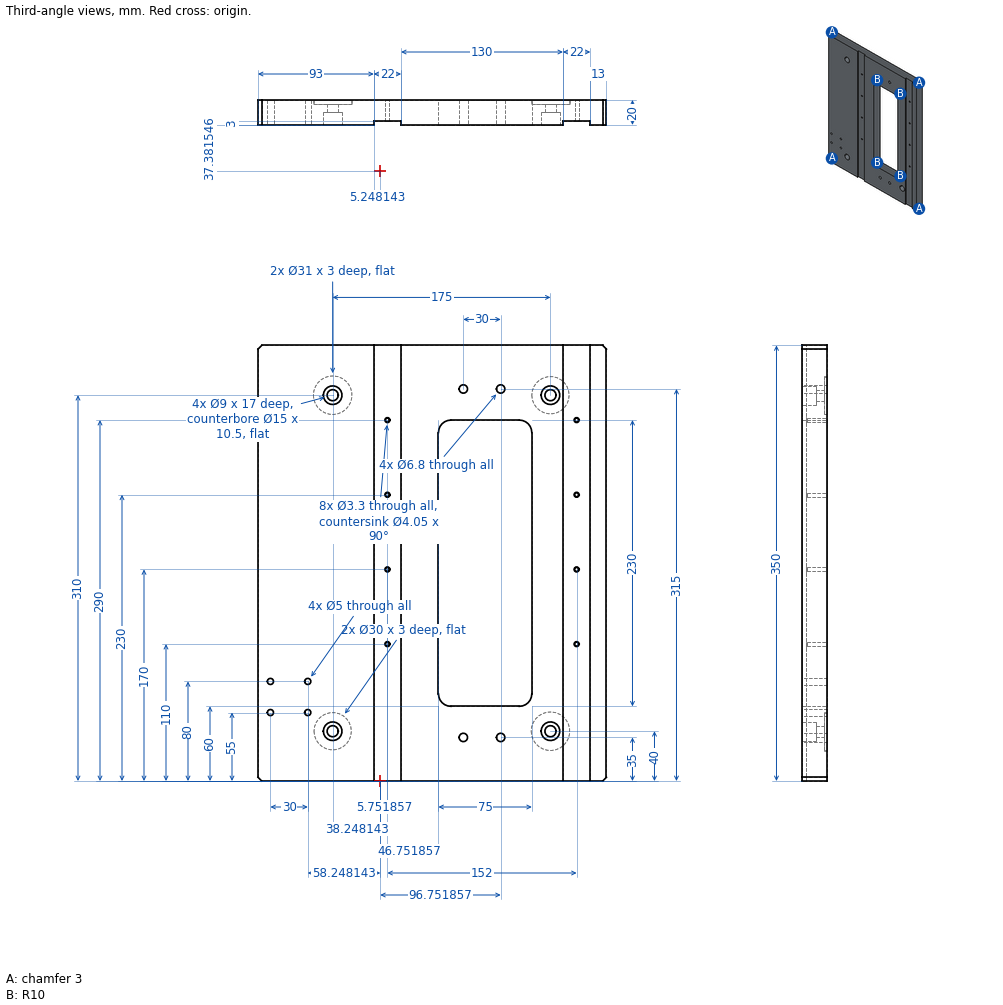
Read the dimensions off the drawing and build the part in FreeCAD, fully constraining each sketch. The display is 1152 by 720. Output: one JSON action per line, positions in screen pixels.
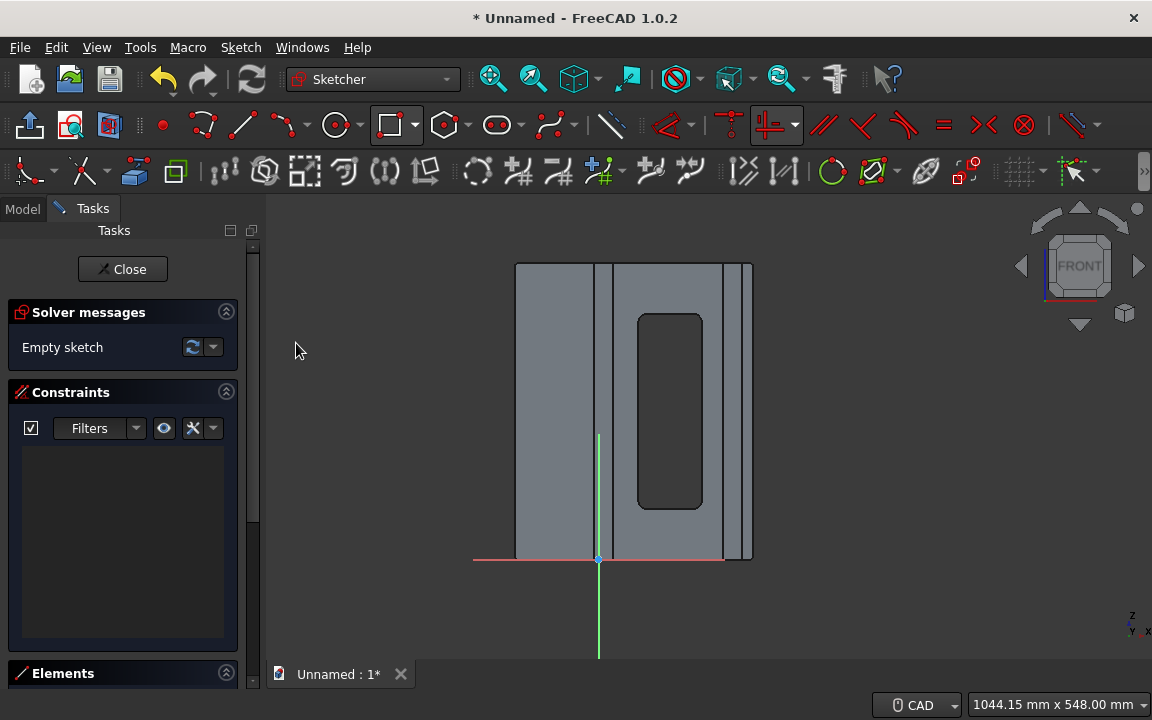
{"action": "left_click", "coordinate": [336, 126]}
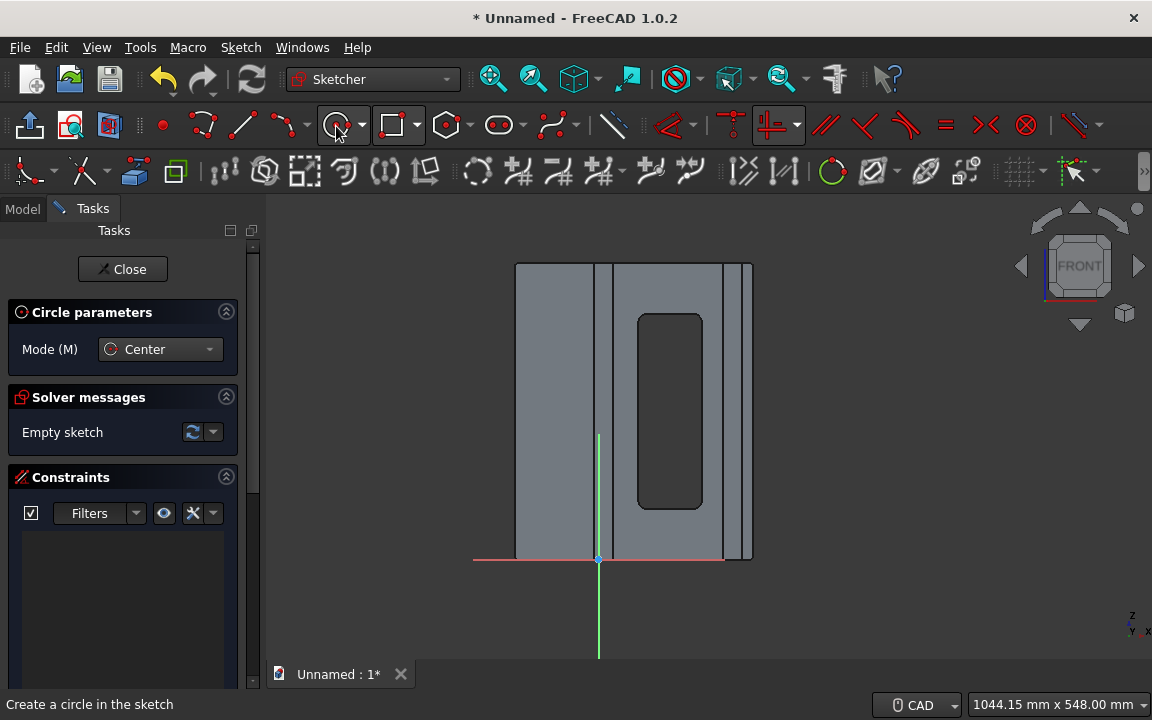
{"action": "scroll", "coordinate": [566, 297], "scroll_direction": "up", "scroll_amount": 9}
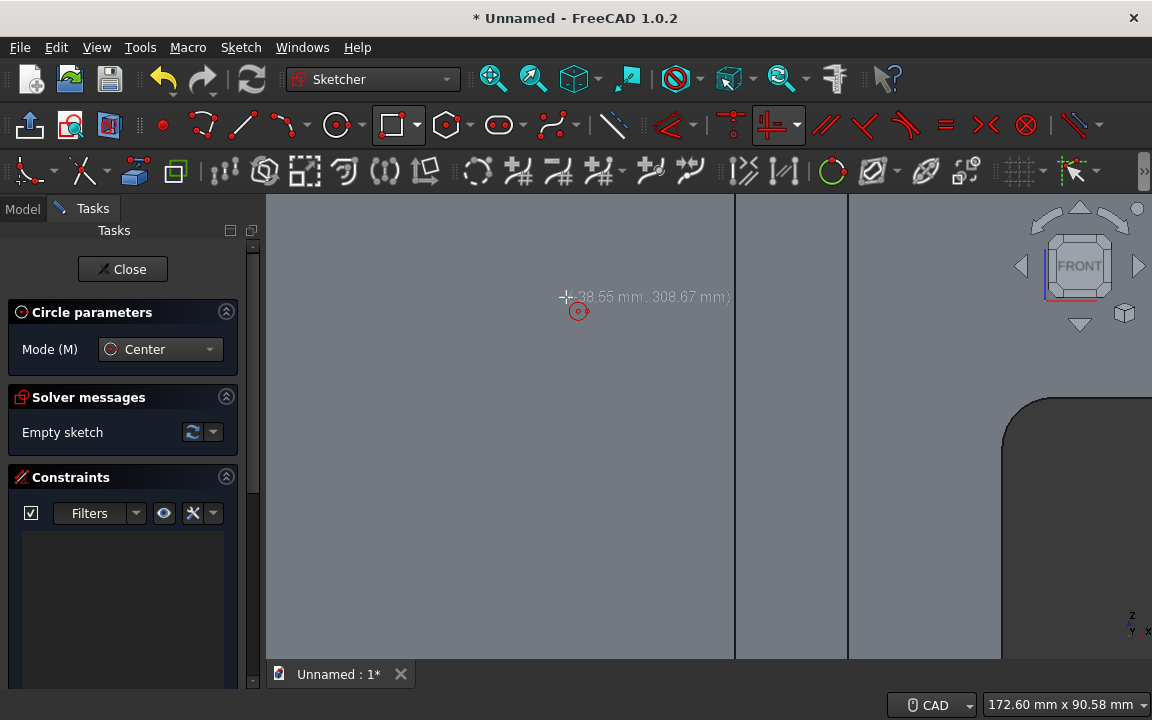
{"action": "scroll", "coordinate": [566, 297], "scroll_direction": "down", "scroll_amount": 9}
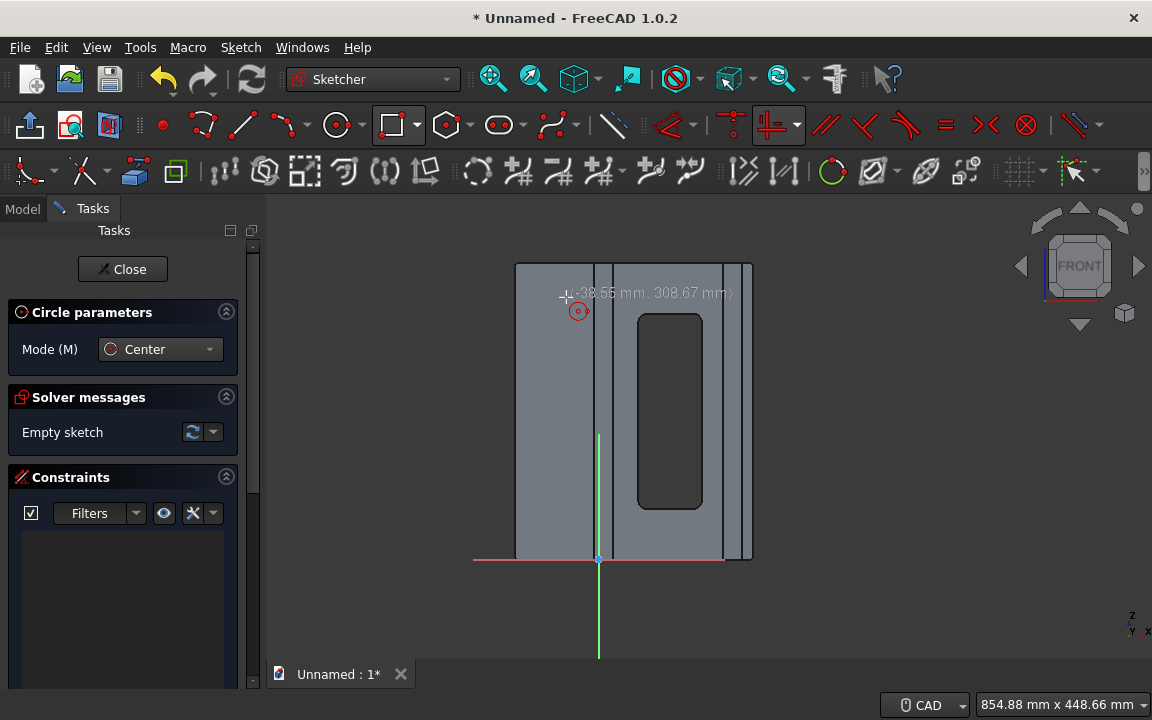
{"action": "left_click", "coordinate": [566, 297]}
{"action": "mouse_move", "coordinate": [569, 294]}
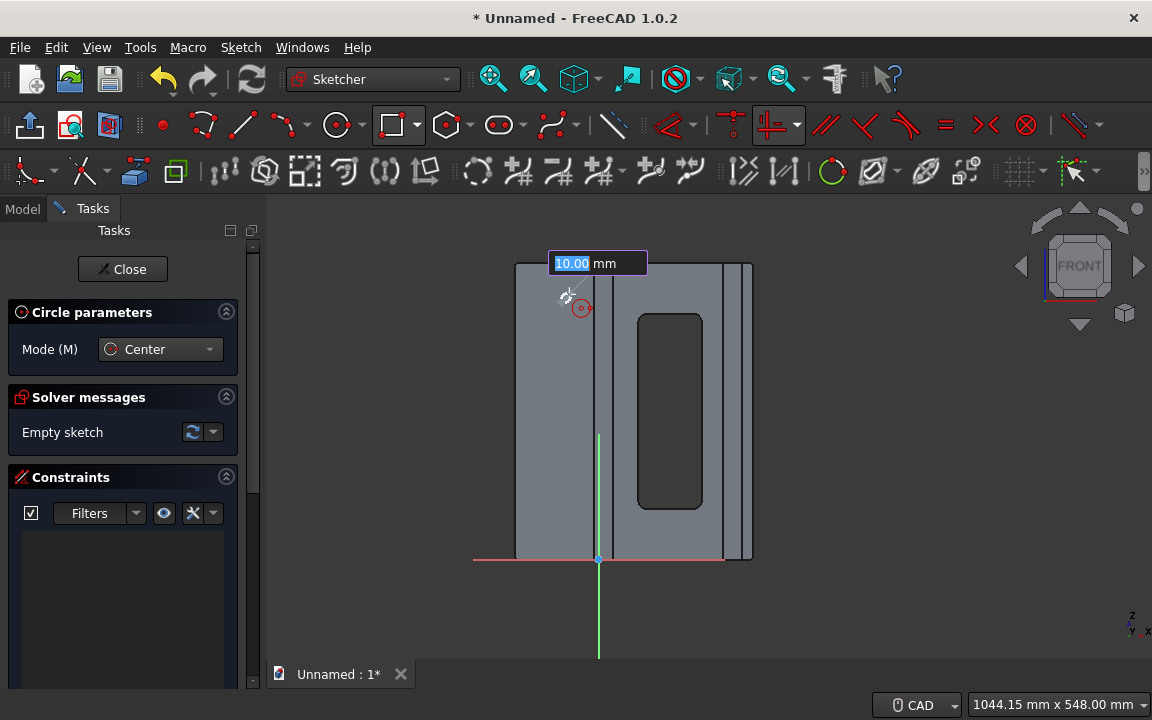
{"action": "type", "text": "9"}
{"action": "key", "text": "Return"}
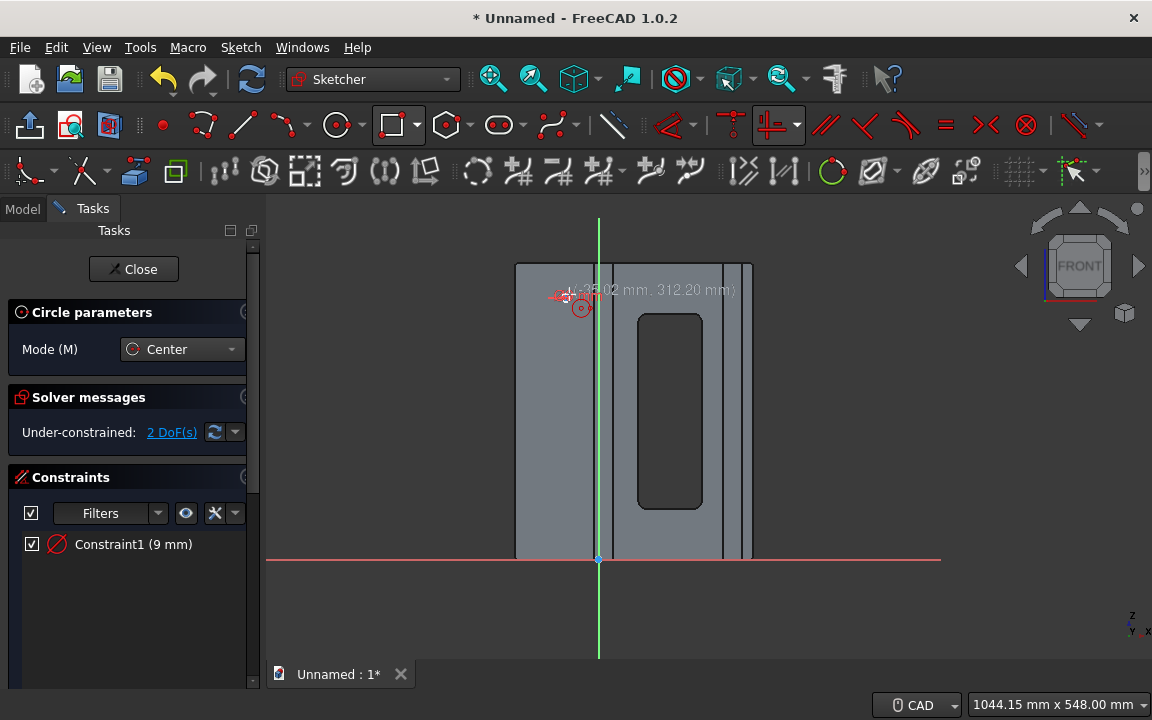
{"action": "scroll", "coordinate": [715, 297], "scroll_direction": "up", "scroll_amount": 9}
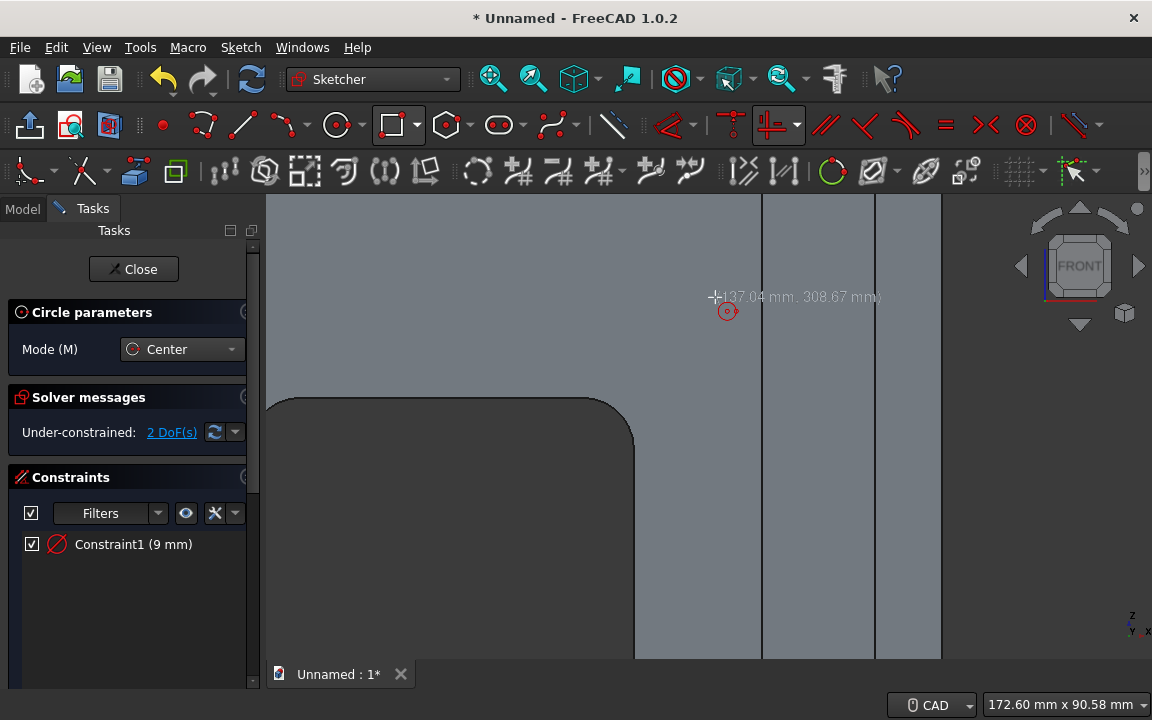
{"action": "scroll", "coordinate": [716, 297], "scroll_direction": "down", "scroll_amount": 9}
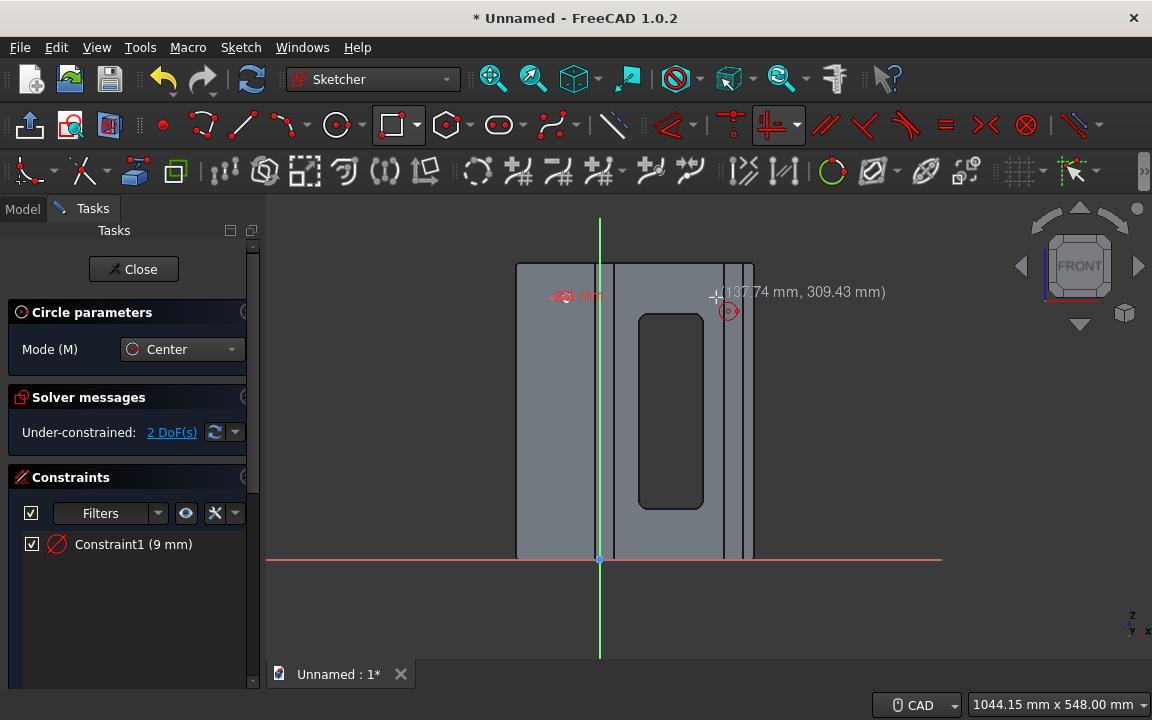
{"action": "left_click", "coordinate": [716, 297]}
{"action": "mouse_move", "coordinate": [718, 294]}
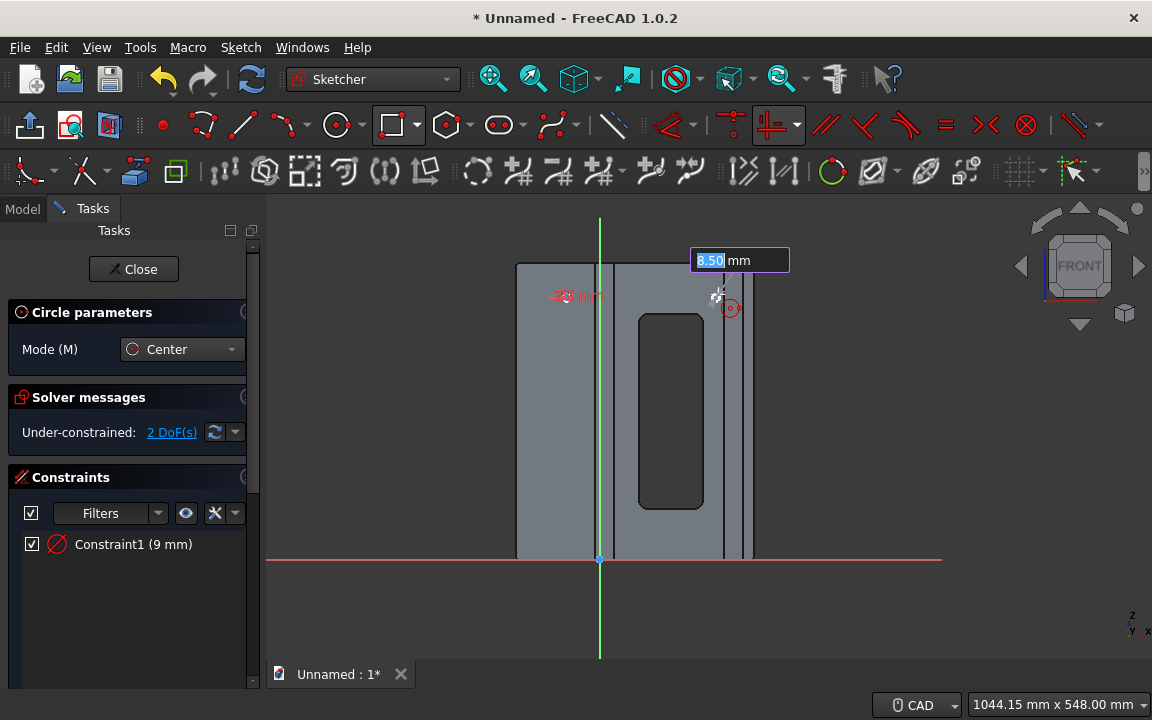
{"action": "type", "text": "9"}
{"action": "key", "text": "Return"}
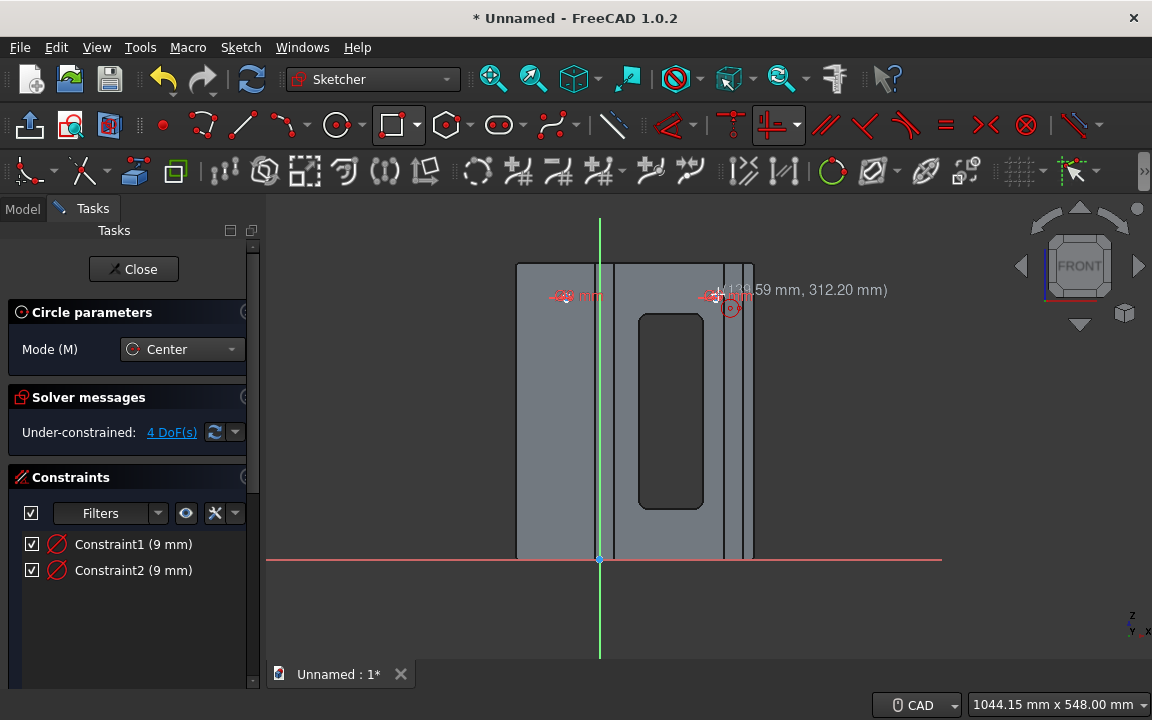
{"action": "scroll", "coordinate": [716, 526], "scroll_direction": "up", "scroll_amount": 9}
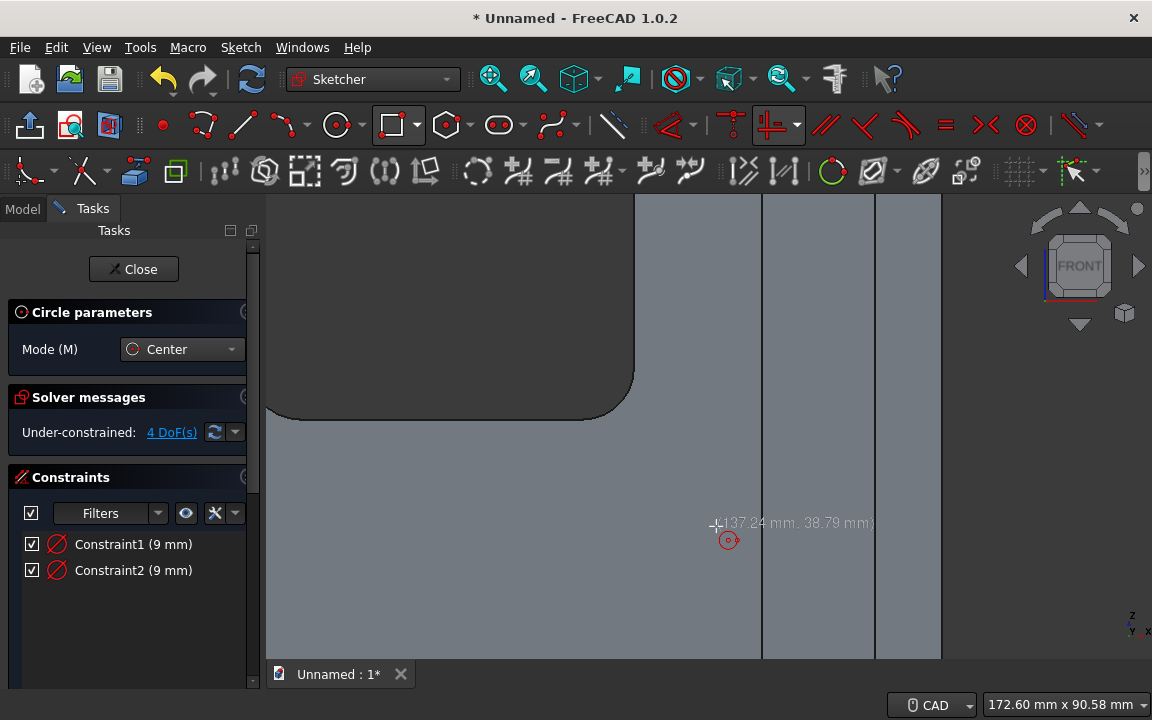
{"action": "scroll", "coordinate": [716, 527], "scroll_direction": "down", "scroll_amount": 9}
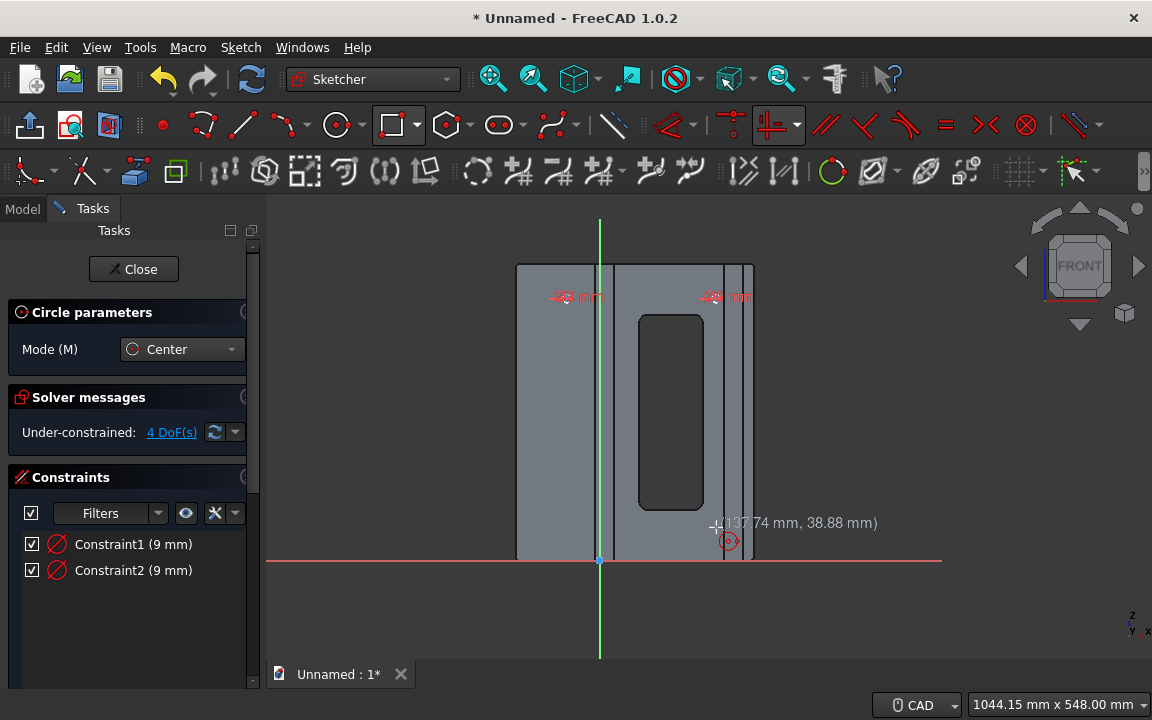
{"action": "left_click", "coordinate": [716, 527]}
{"action": "mouse_move", "coordinate": [718, 524]}